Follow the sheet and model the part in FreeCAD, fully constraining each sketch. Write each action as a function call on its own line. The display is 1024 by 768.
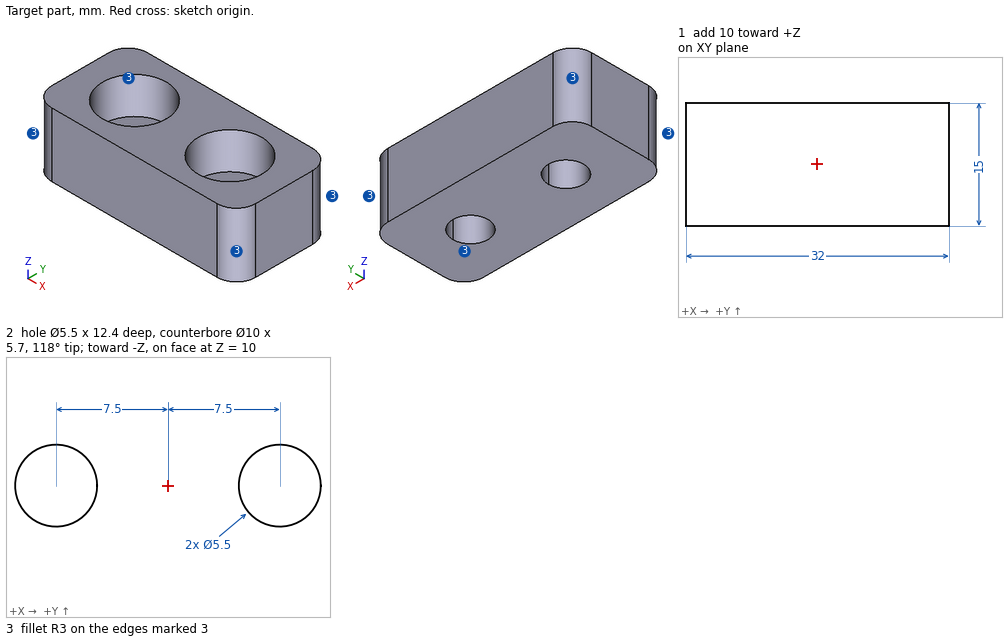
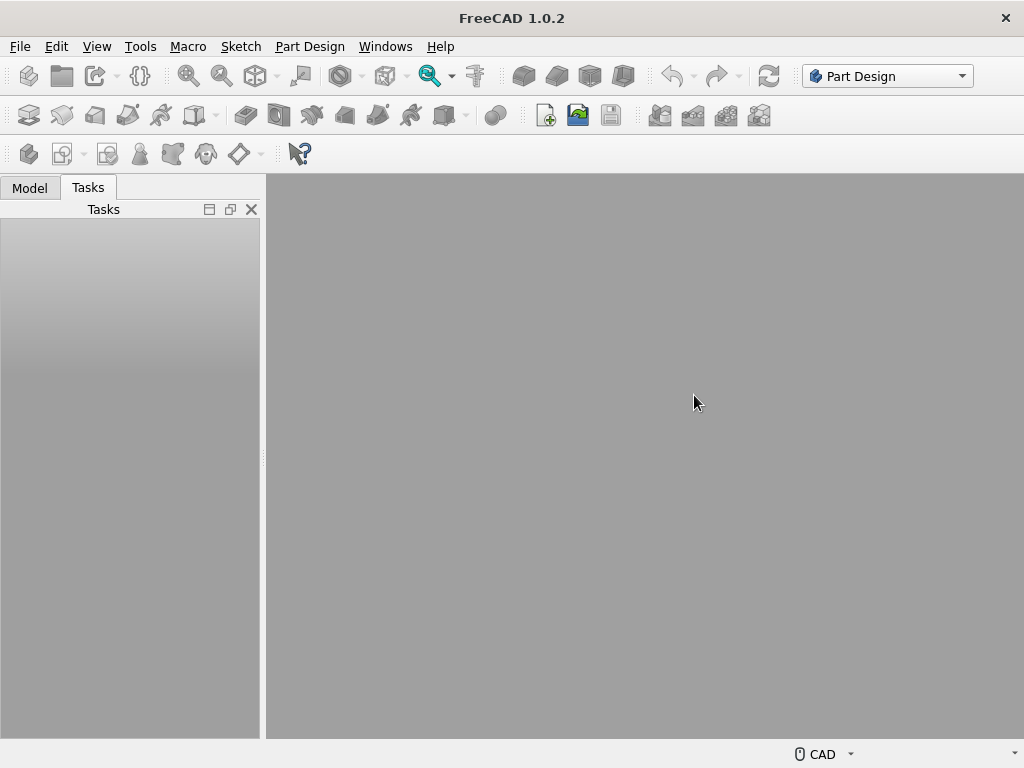
key(ctrl+n)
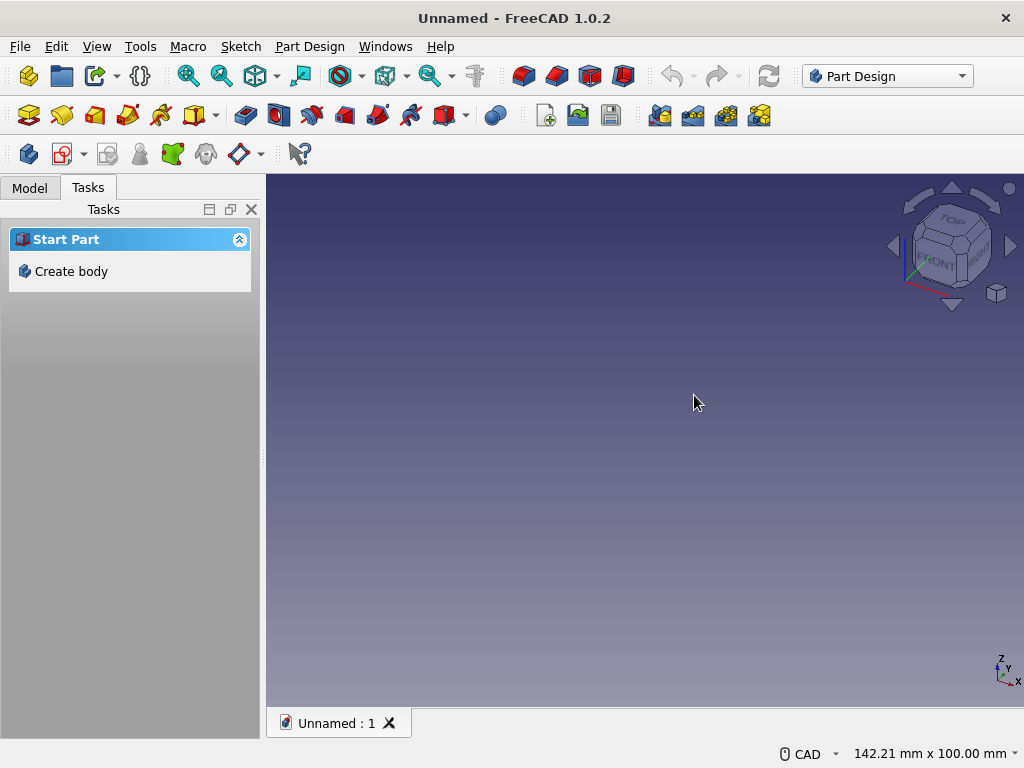
click(62, 154)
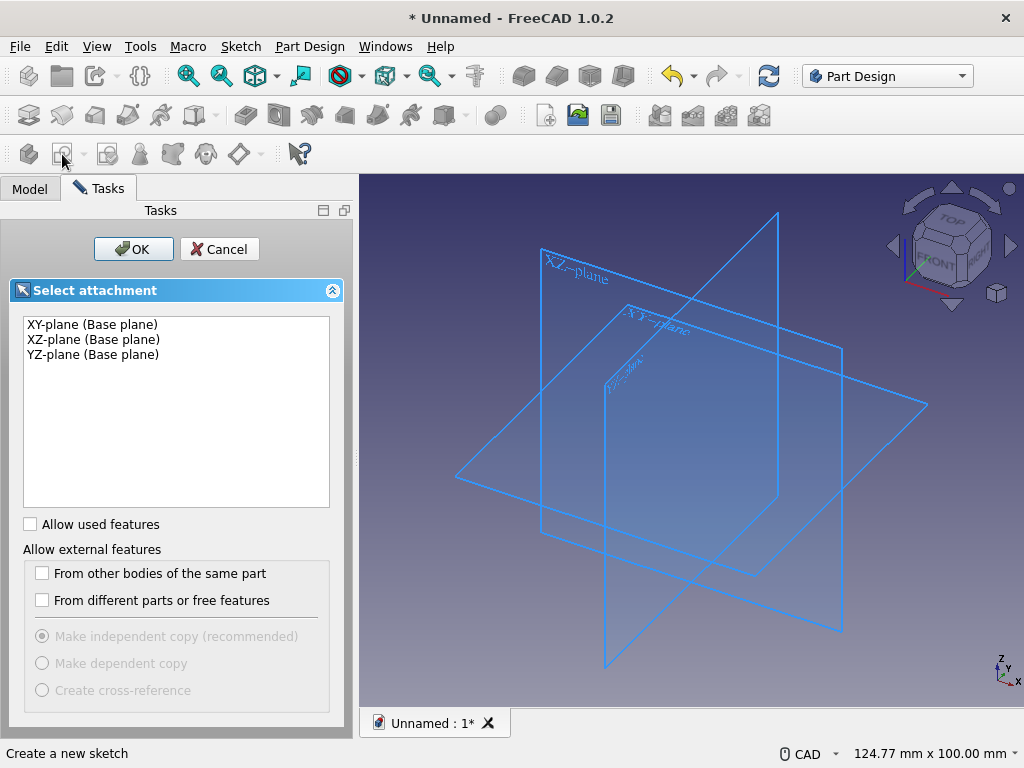
click(84, 324)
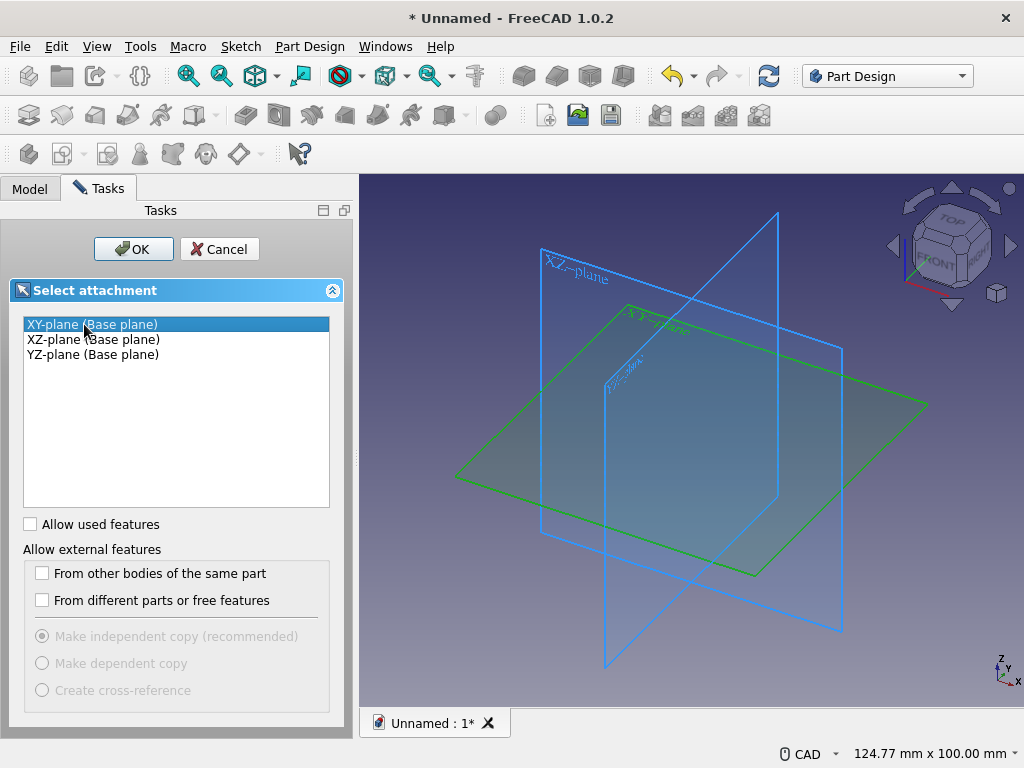
click(134, 249)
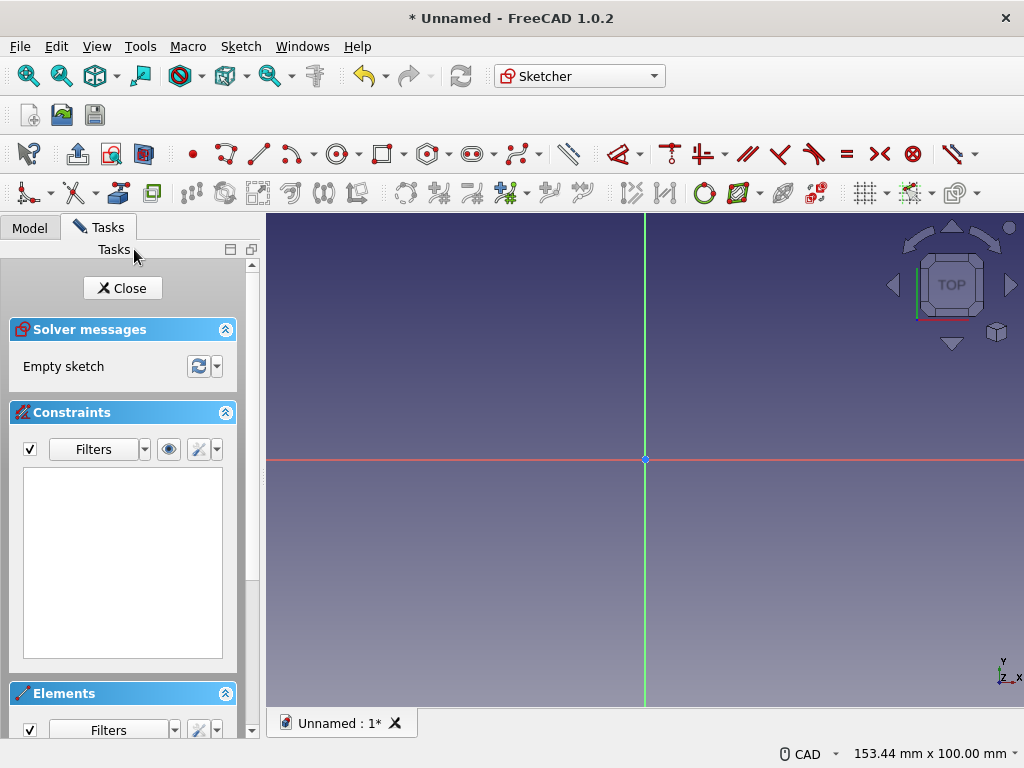
scroll(685, 460, up, 5)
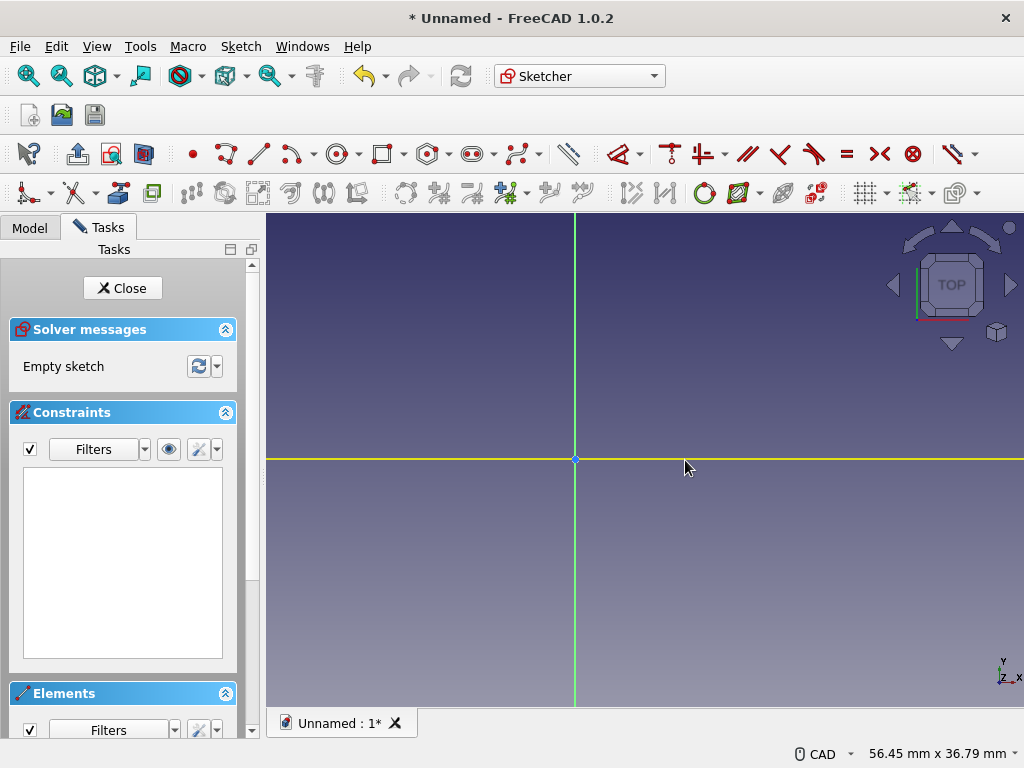
key(g)
key(v)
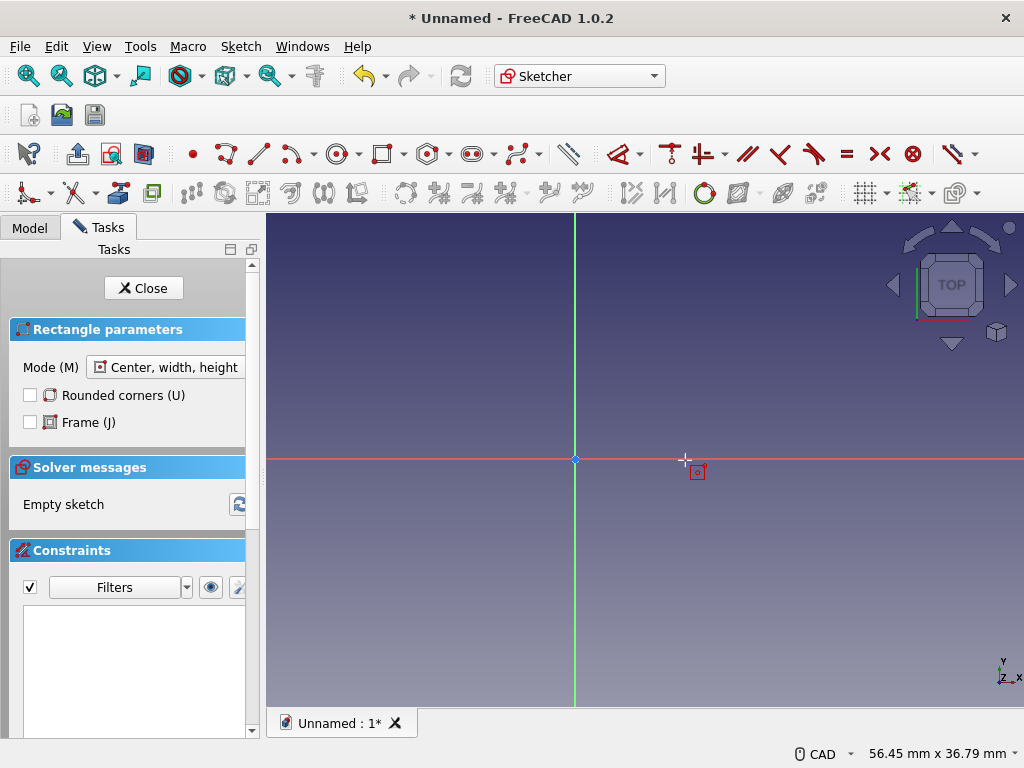
click(575, 459)
move(790, 358)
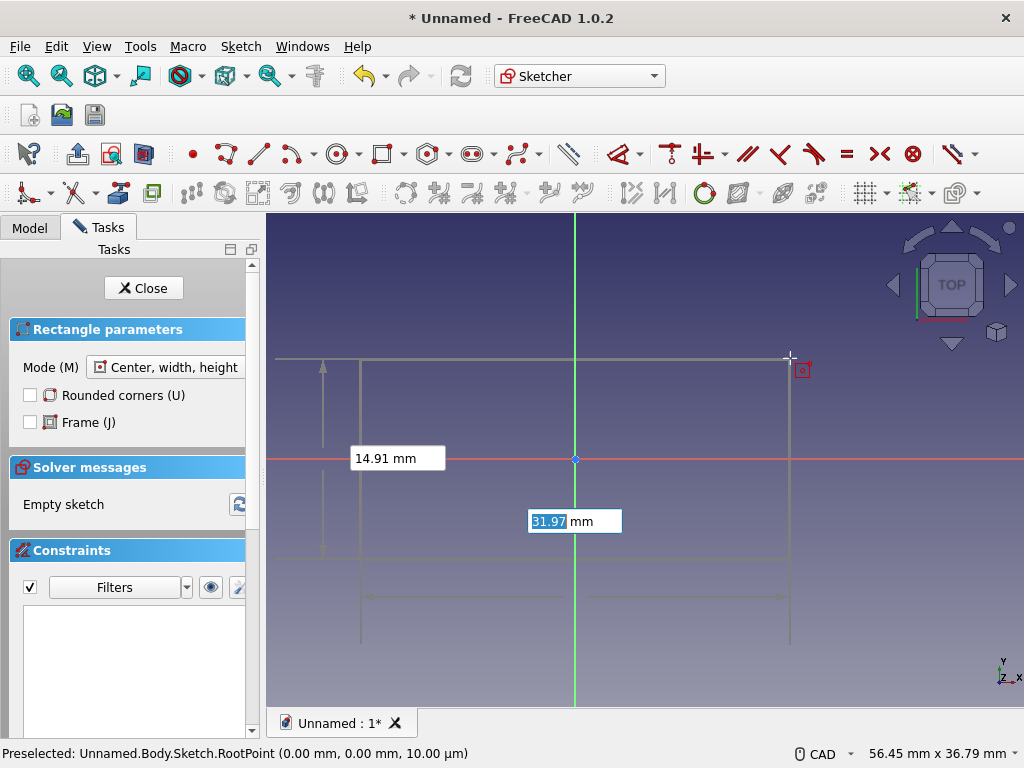
text(32)
key(Tab)
text(15)
key(Return)
key(Escape)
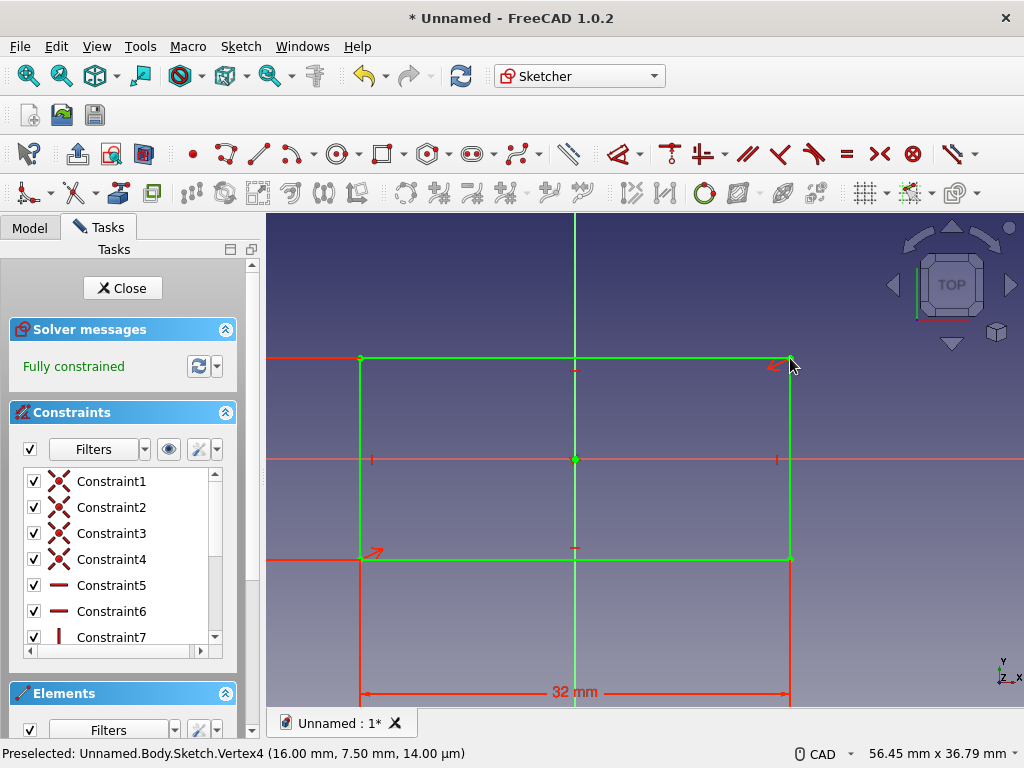
click(123, 288)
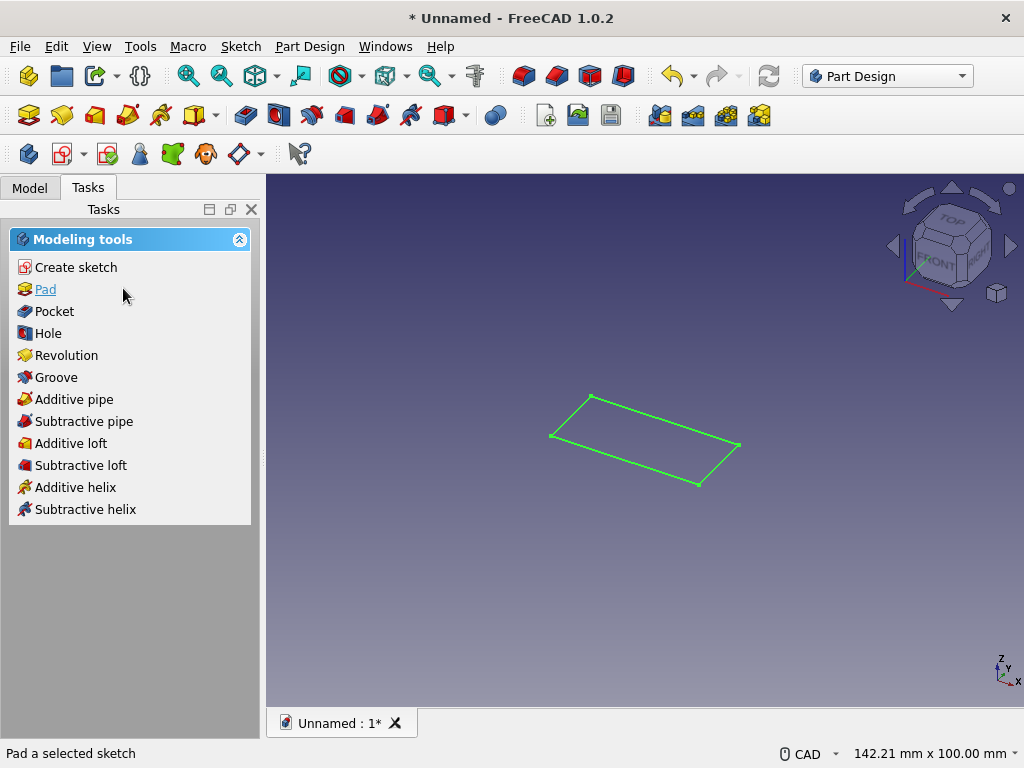
click(29, 116)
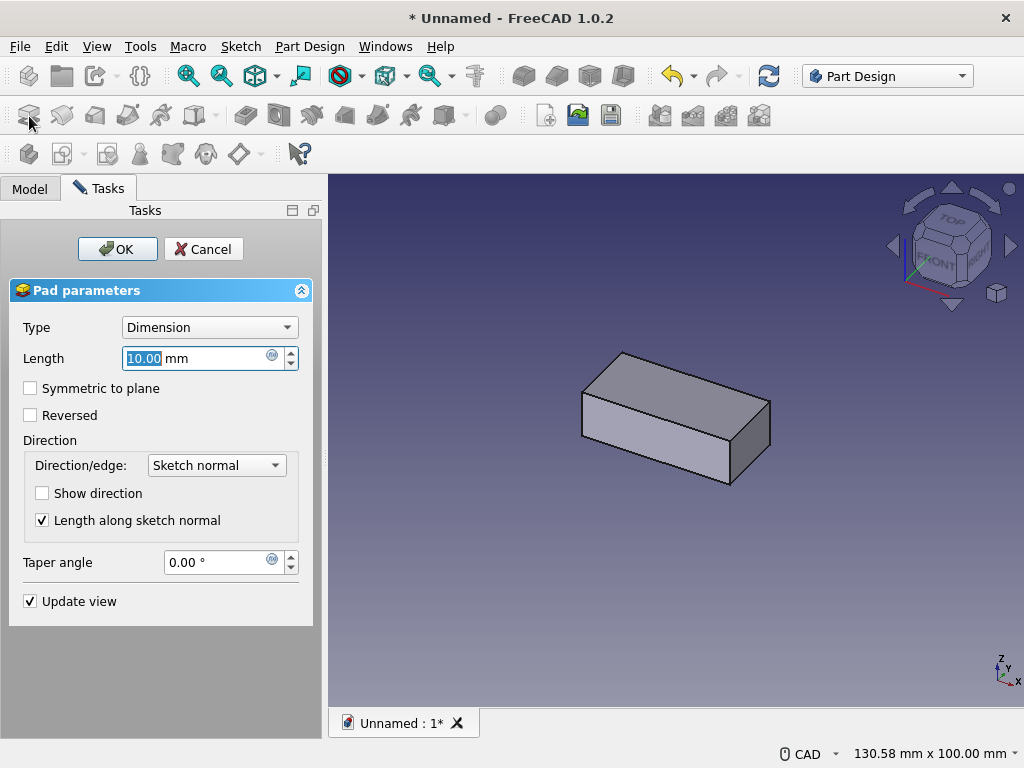
text(10)
key(Tab)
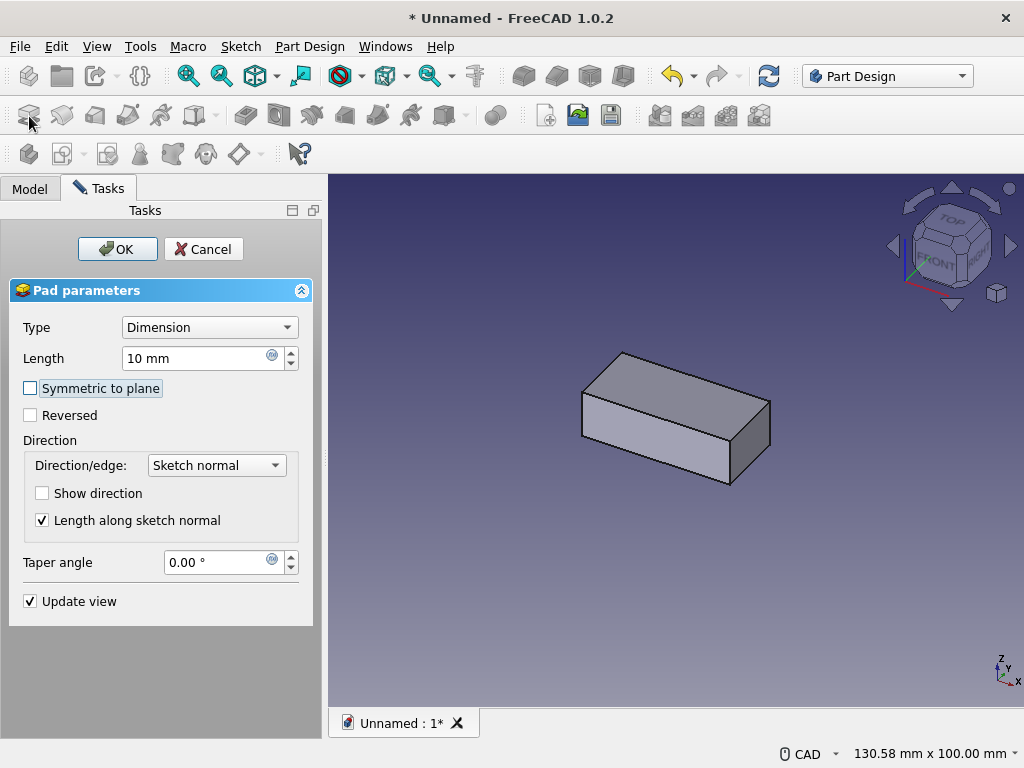
click(118, 249)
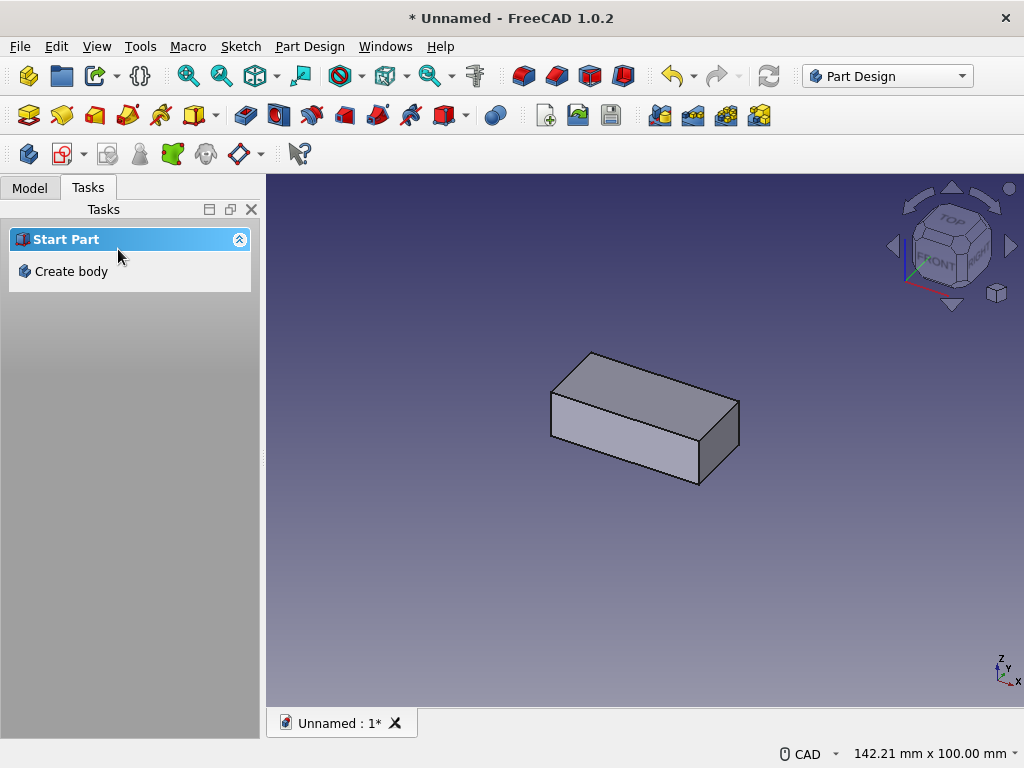
key(v)
key(f)